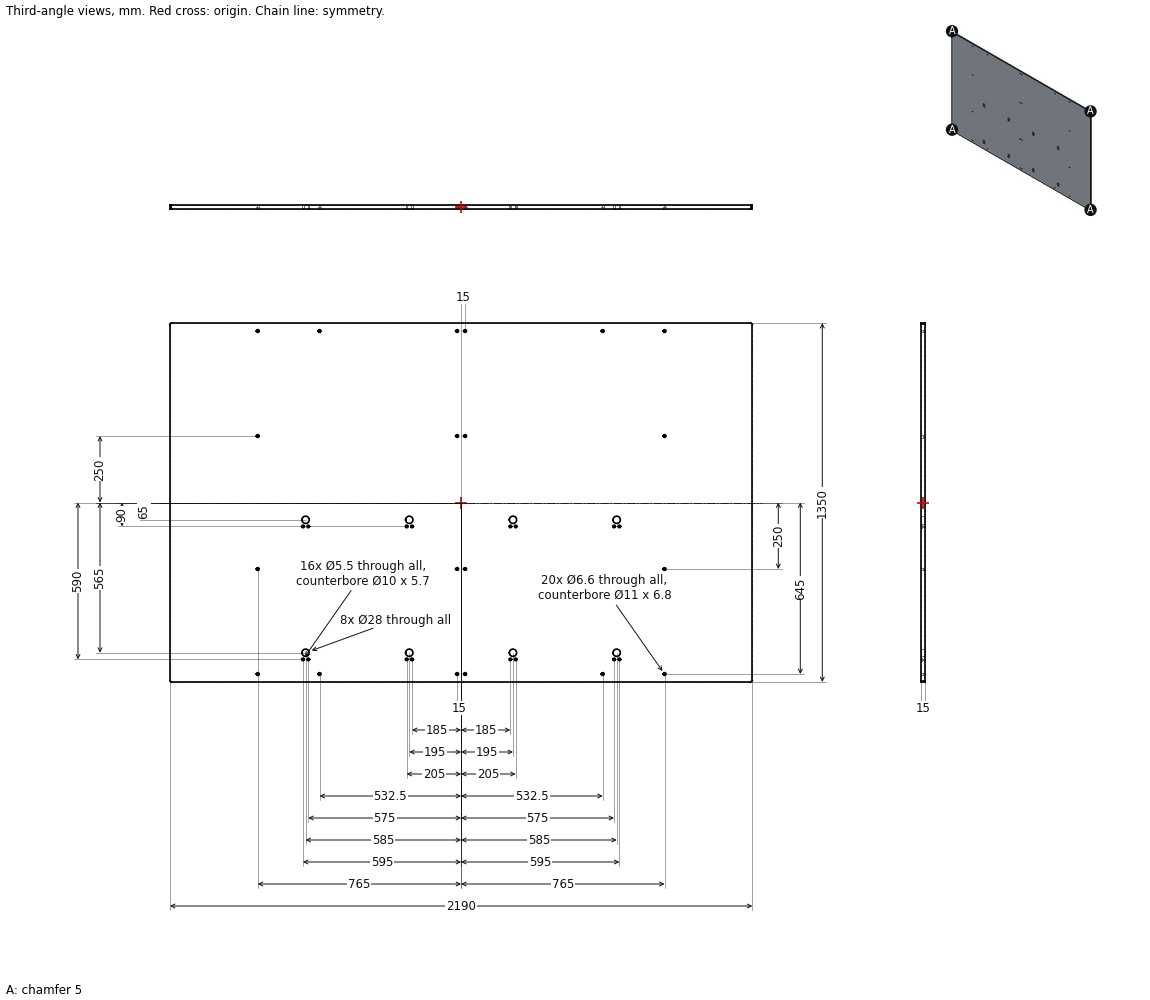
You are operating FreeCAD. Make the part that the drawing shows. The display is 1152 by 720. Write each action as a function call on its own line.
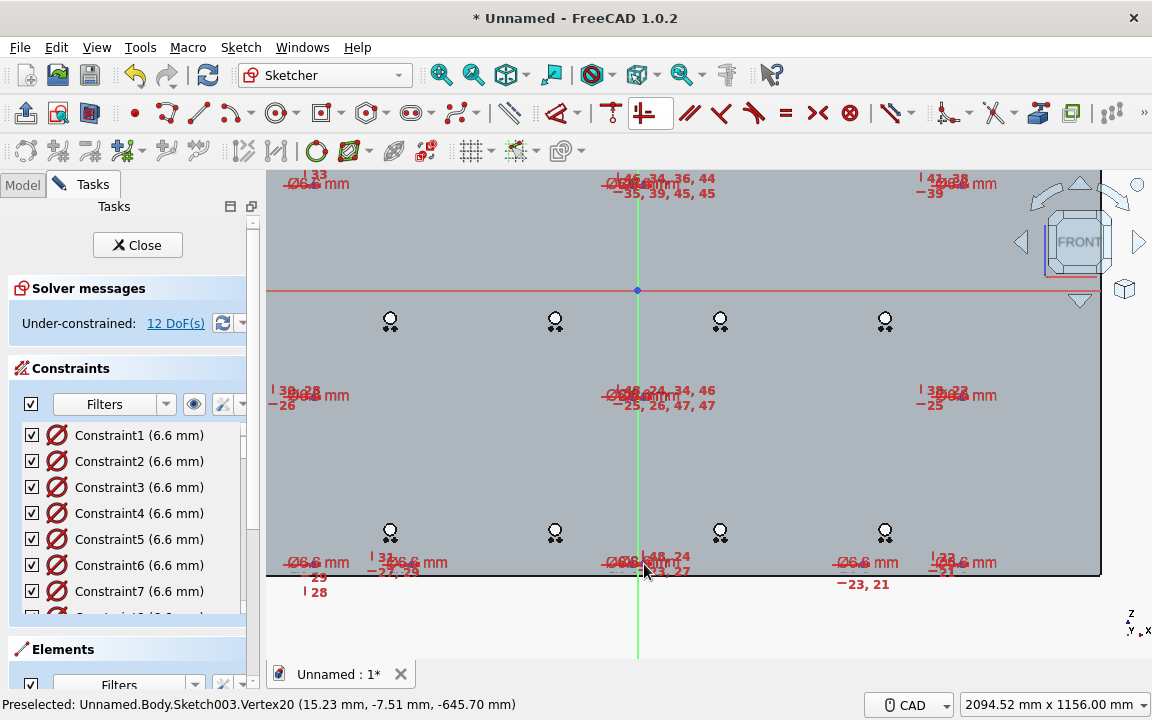
click(632, 565)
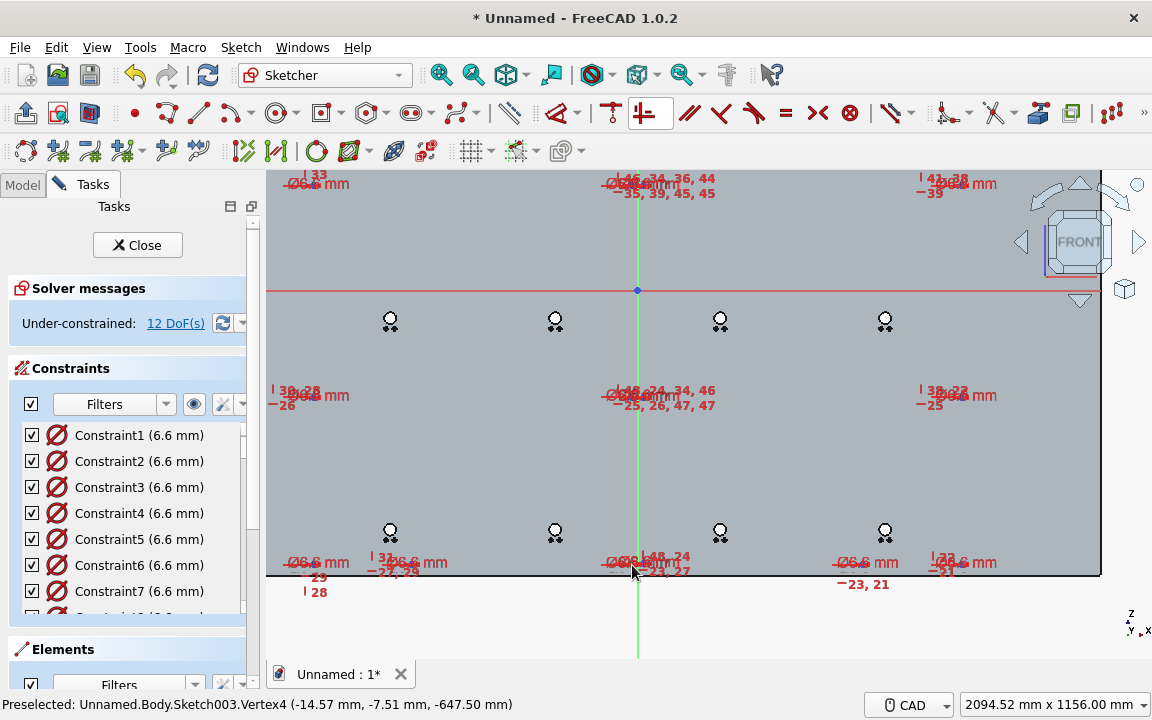
scroll(644, 564, up, 4)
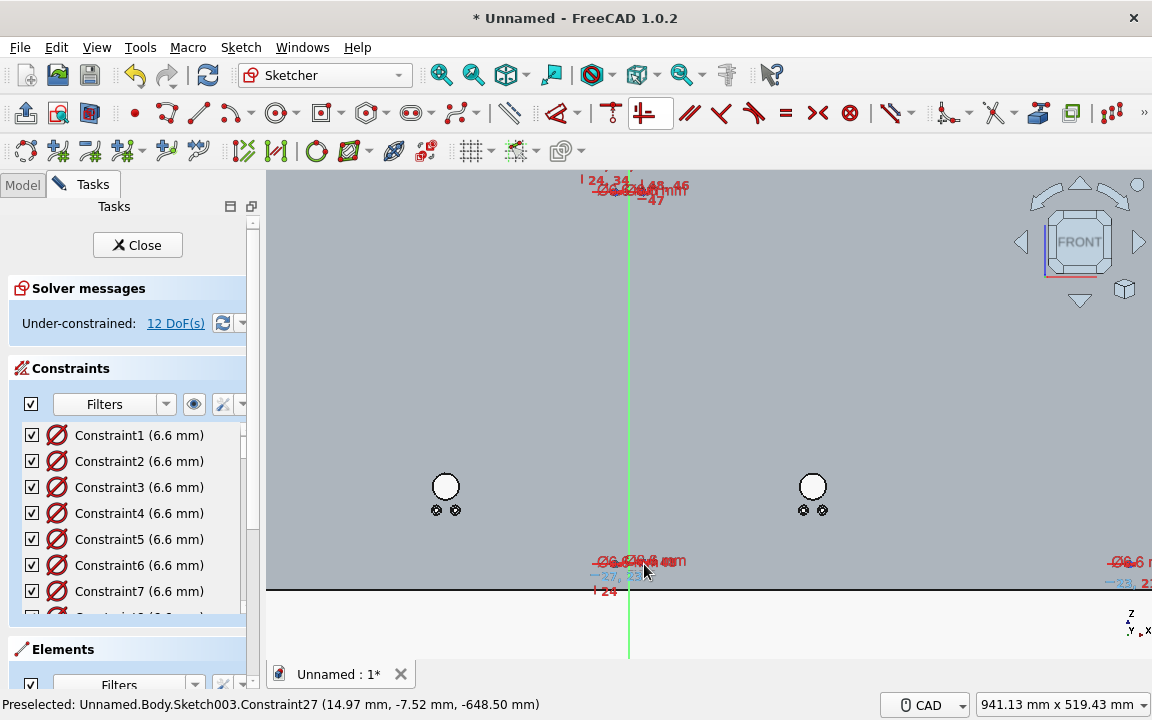
click(643, 563)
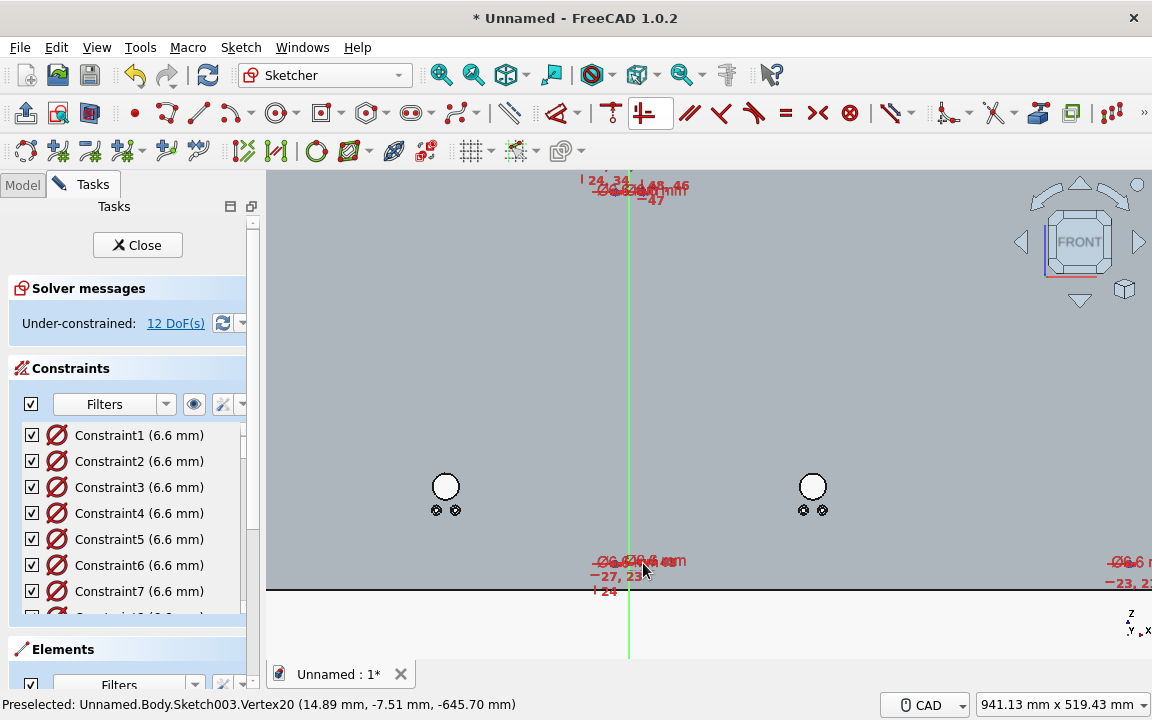
key(h)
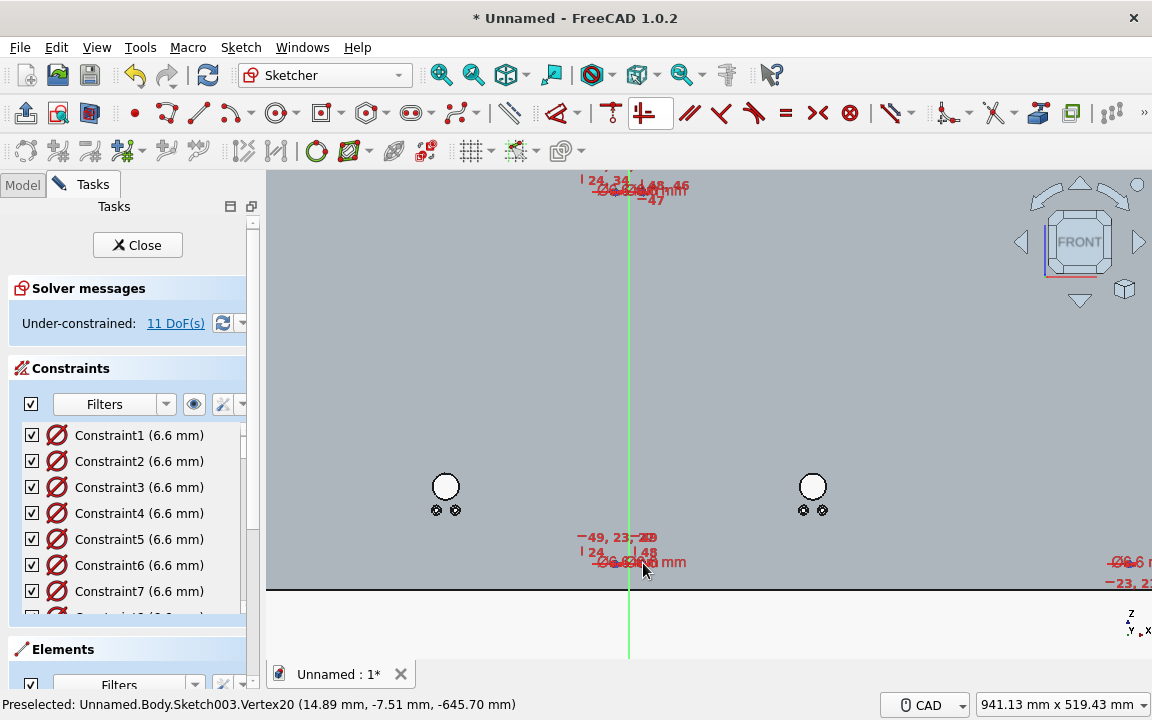
scroll(644, 565, down, 7)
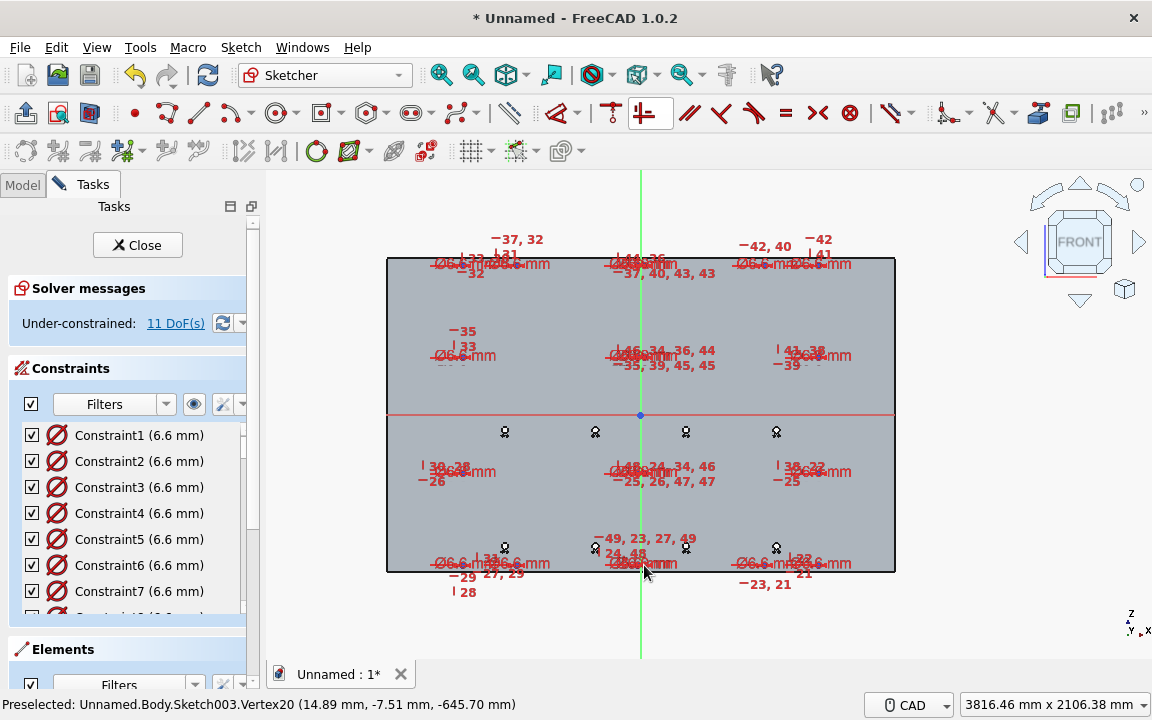
click(764, 565)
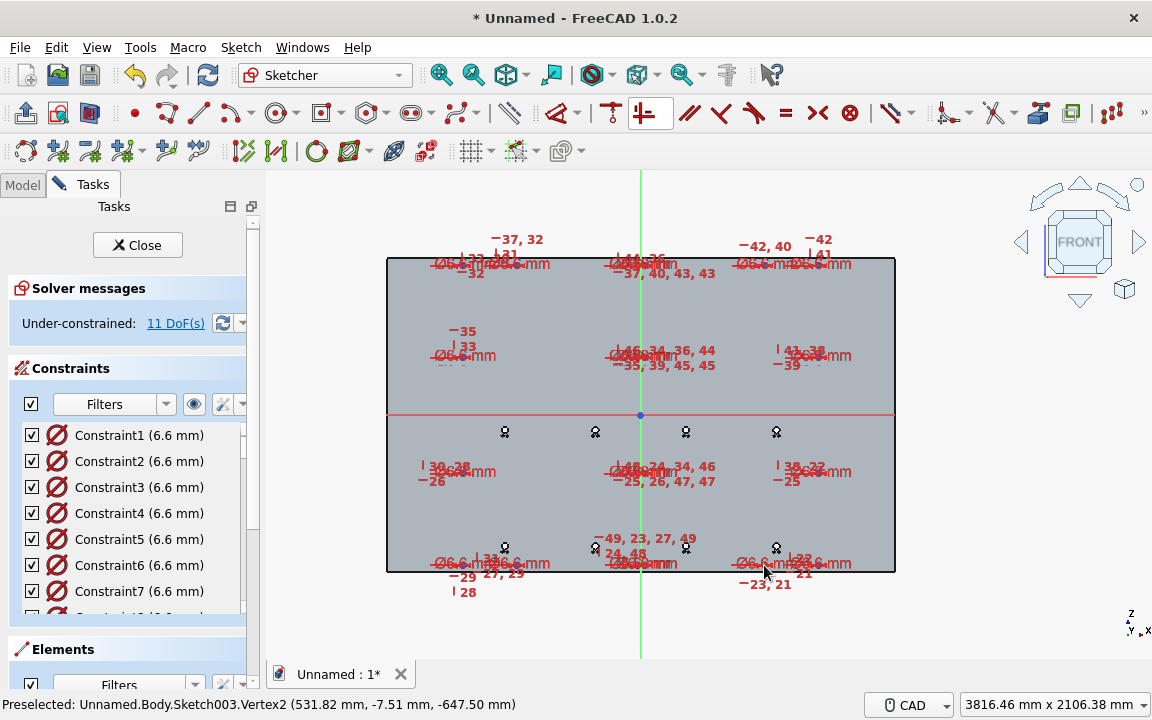
click(765, 266)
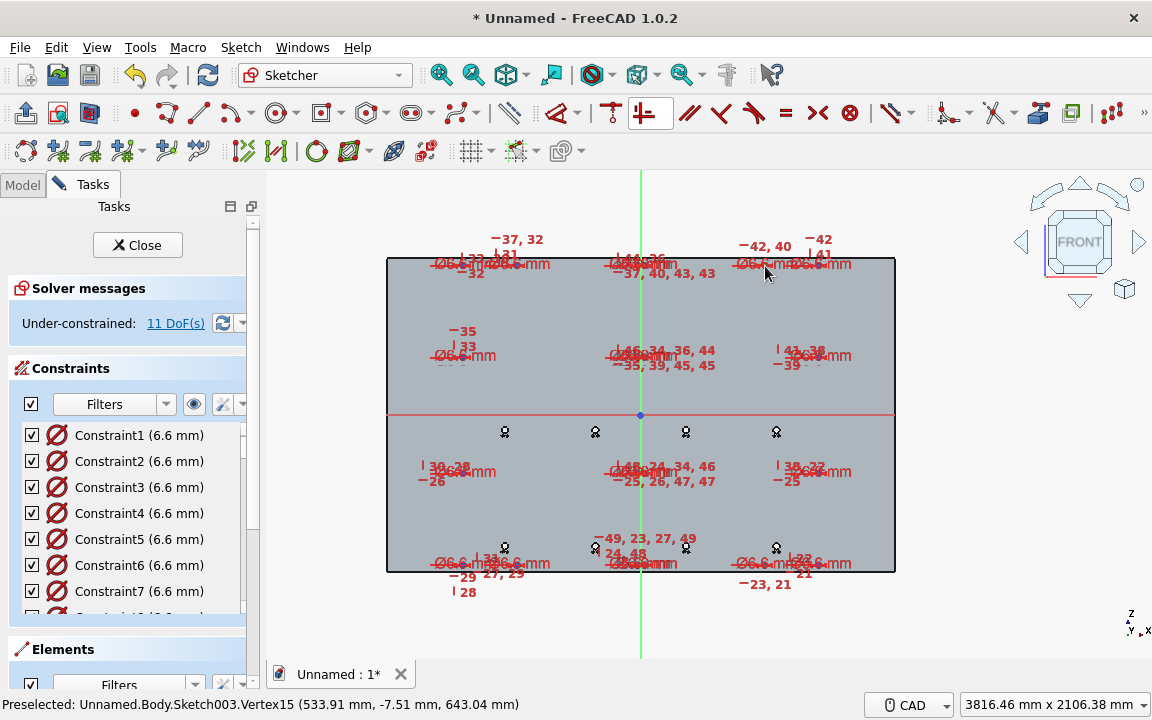
click(393, 415)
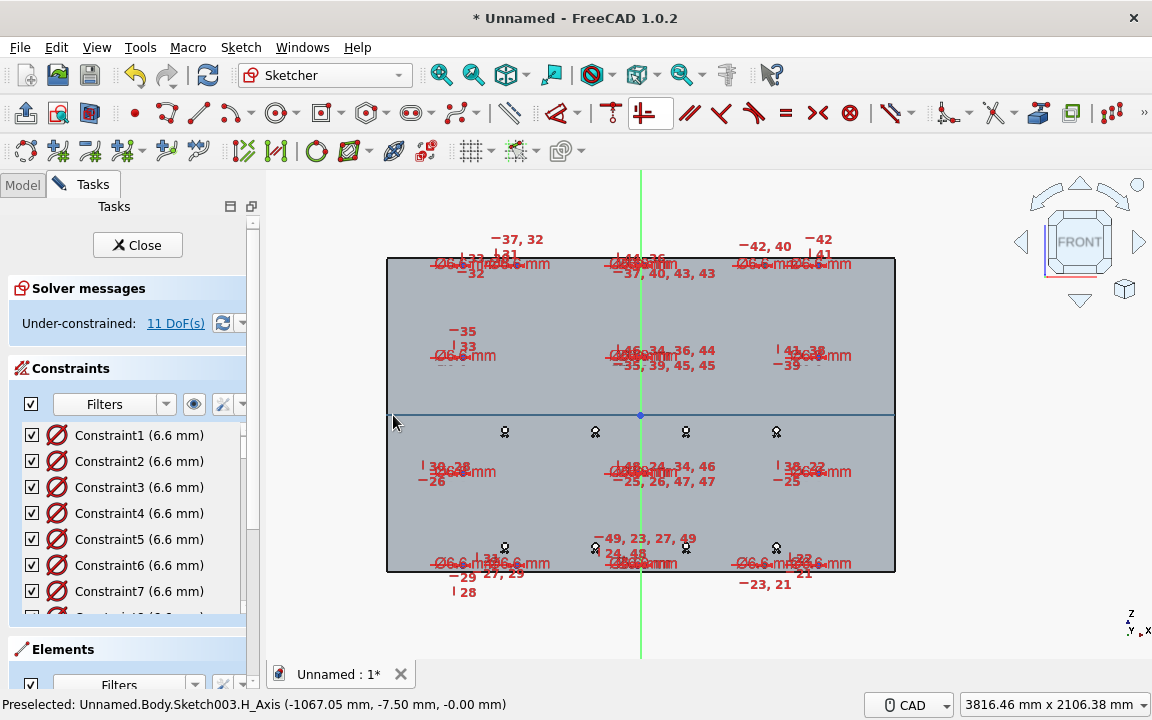
key(s)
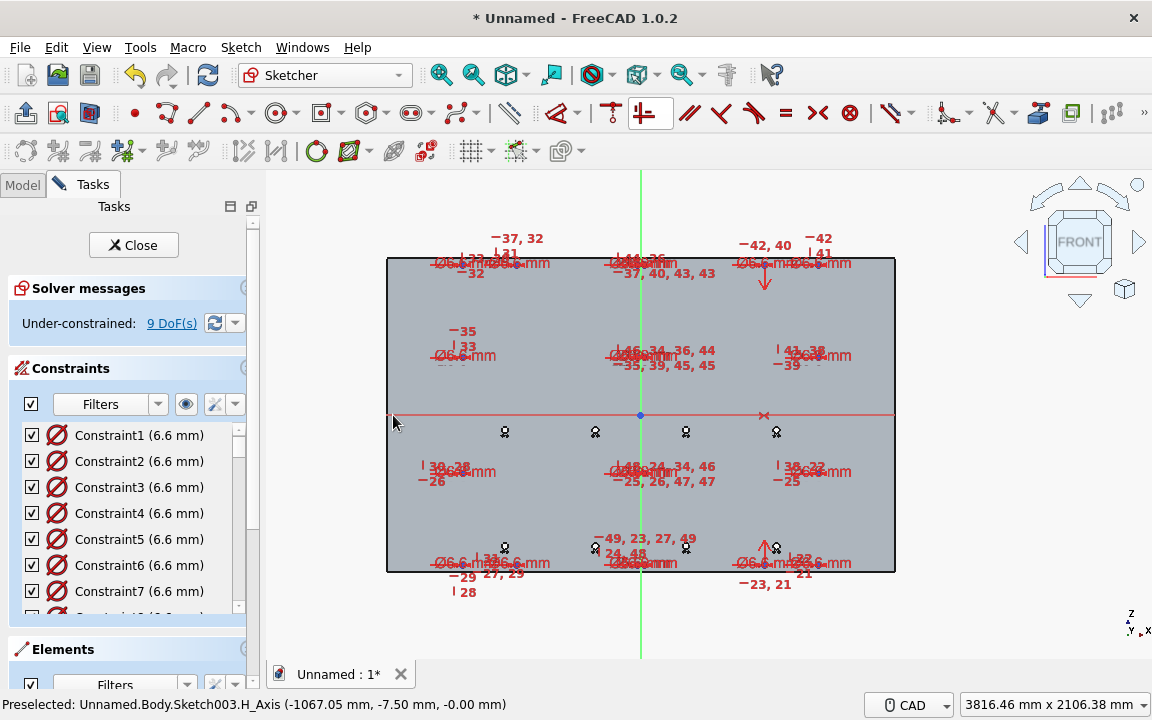
click(556, 114)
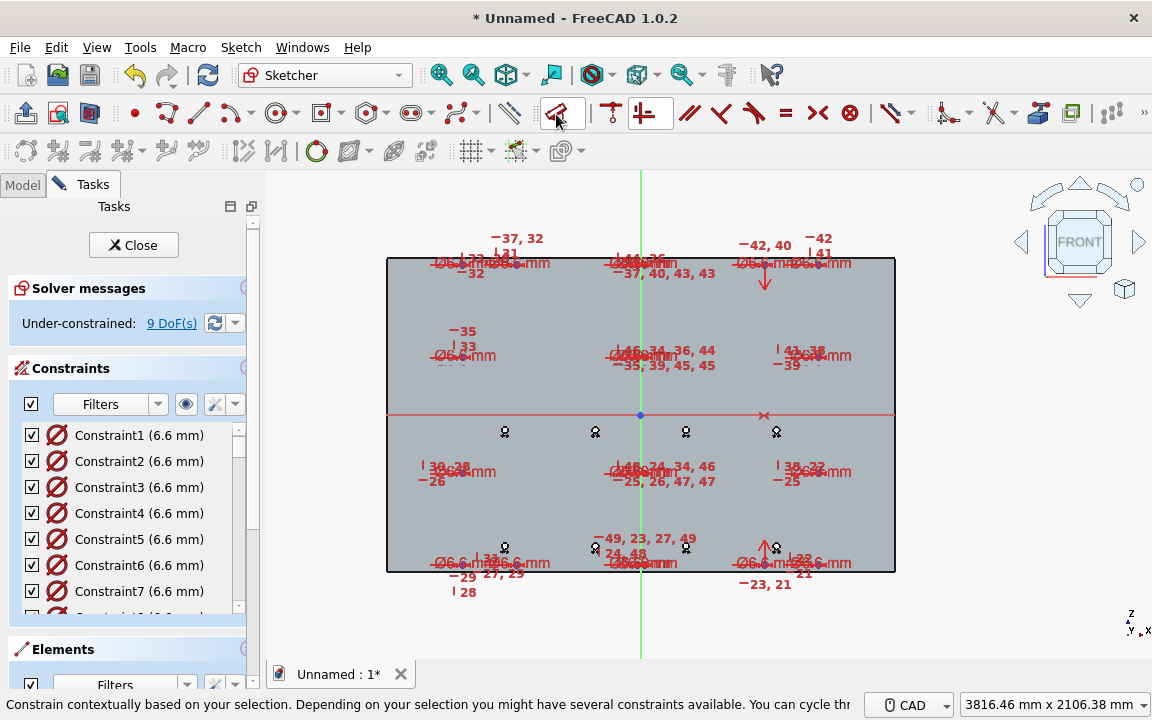
scroll(637, 565, up, 13)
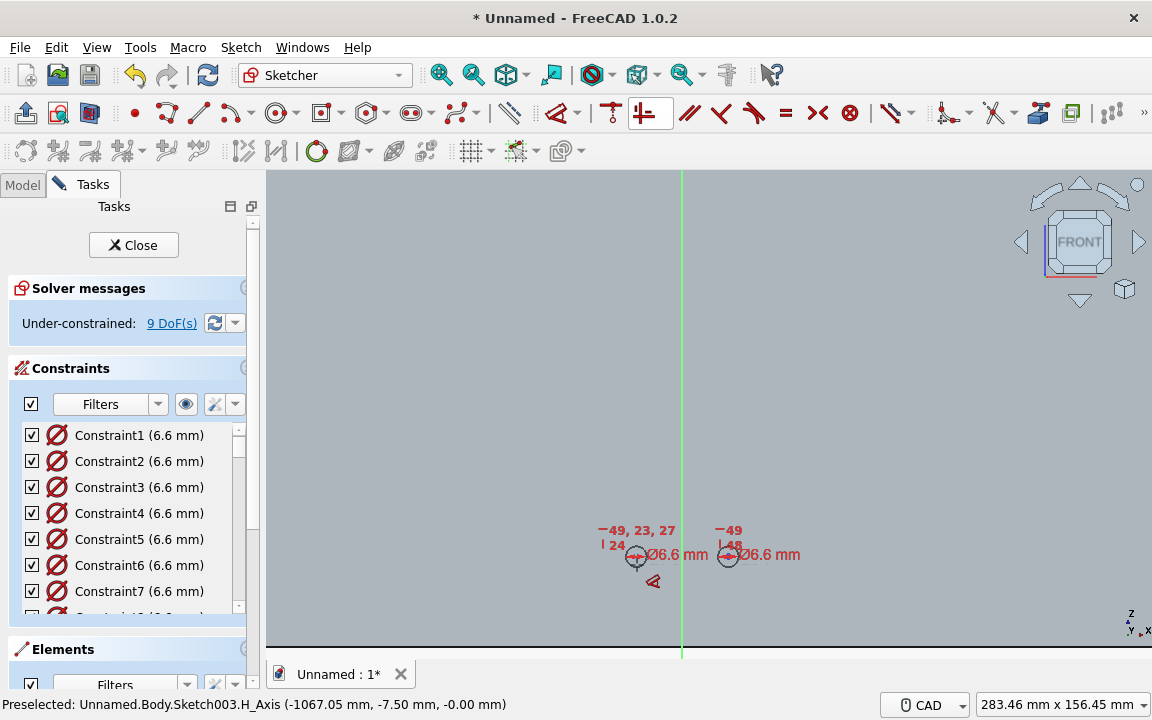
click(636, 557)
click(659, 591)